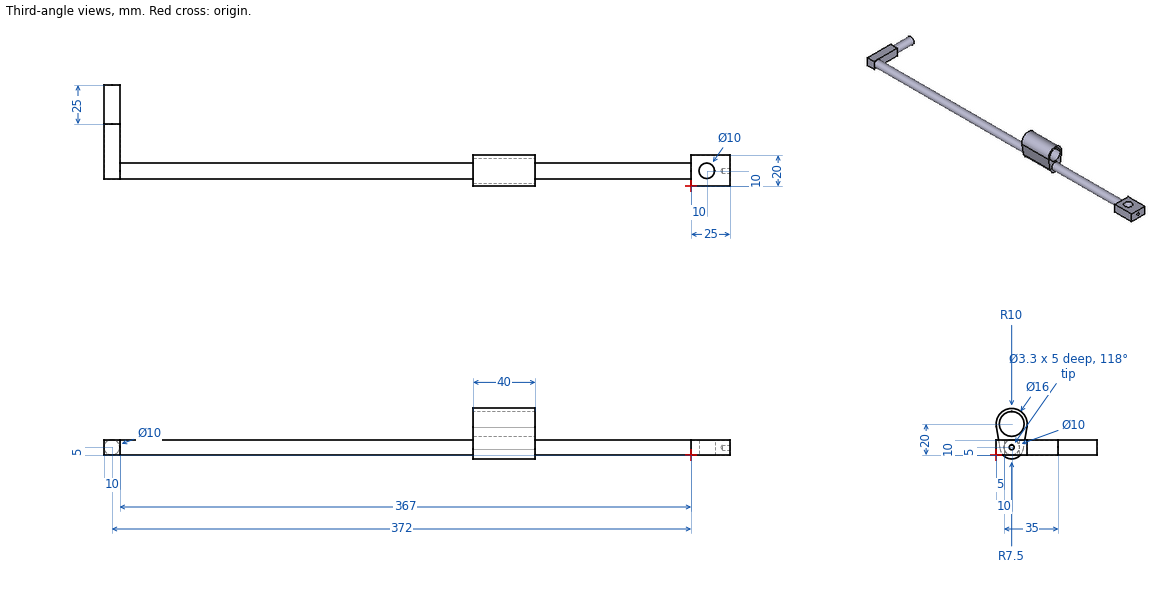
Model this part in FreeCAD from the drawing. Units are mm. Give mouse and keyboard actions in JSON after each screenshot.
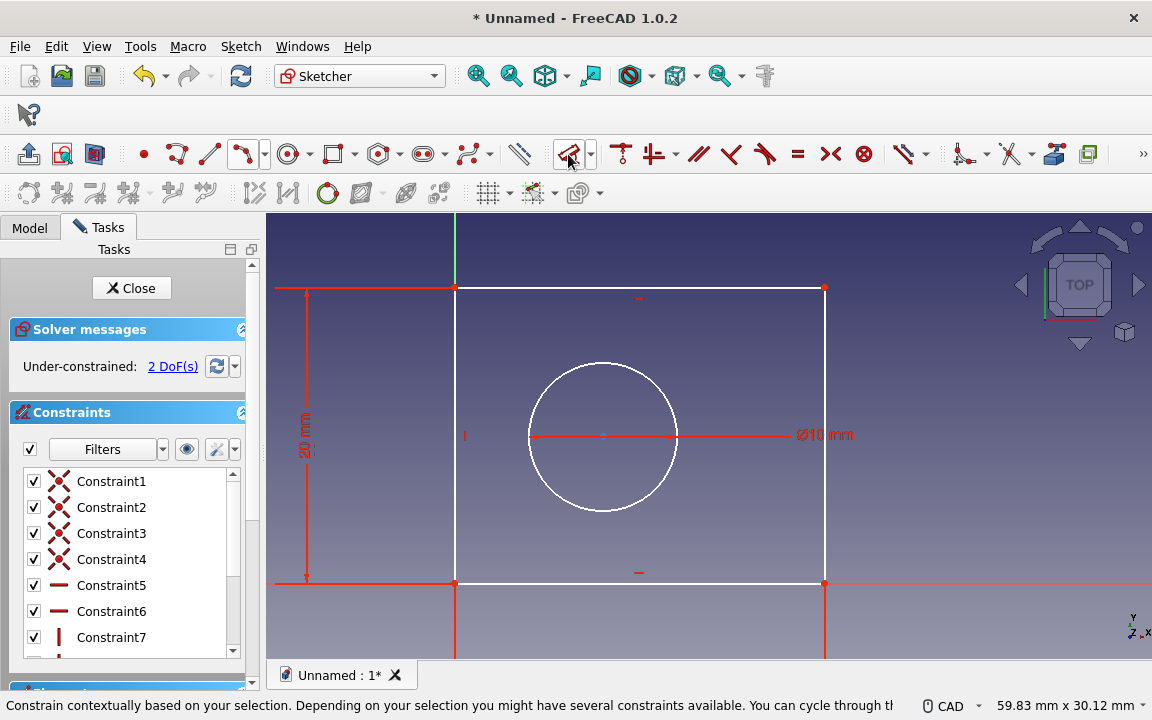
{"action": "left_click", "coordinate": [603, 437]}
{"action": "left_click", "coordinate": [529, 618]}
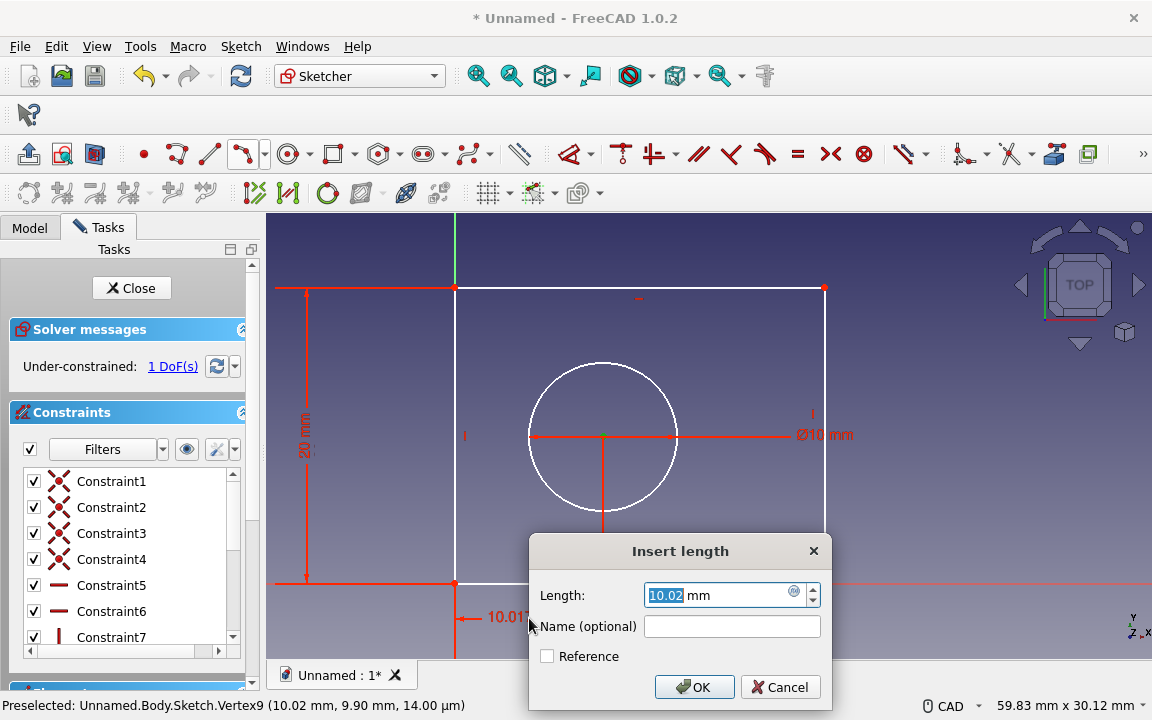
{"action": "type", "text": "10"}
{"action": "key", "text": "Return"}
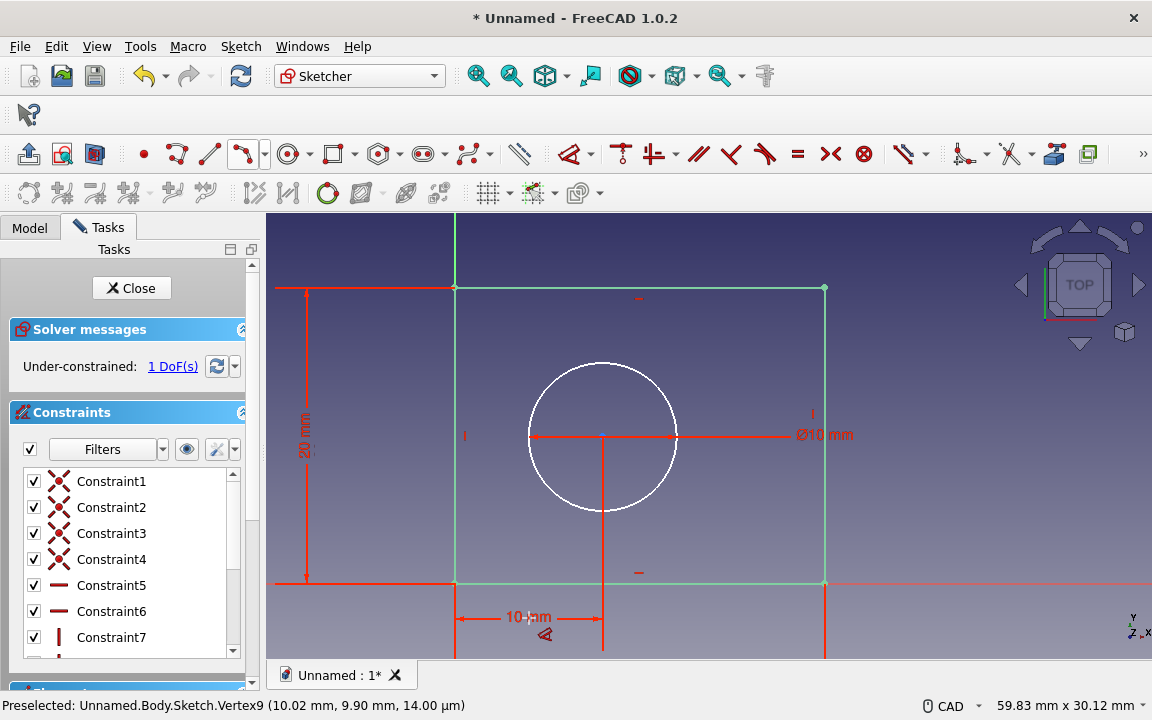
{"action": "left_click", "coordinate": [603, 437]}
{"action": "left_click", "coordinate": [421, 510]}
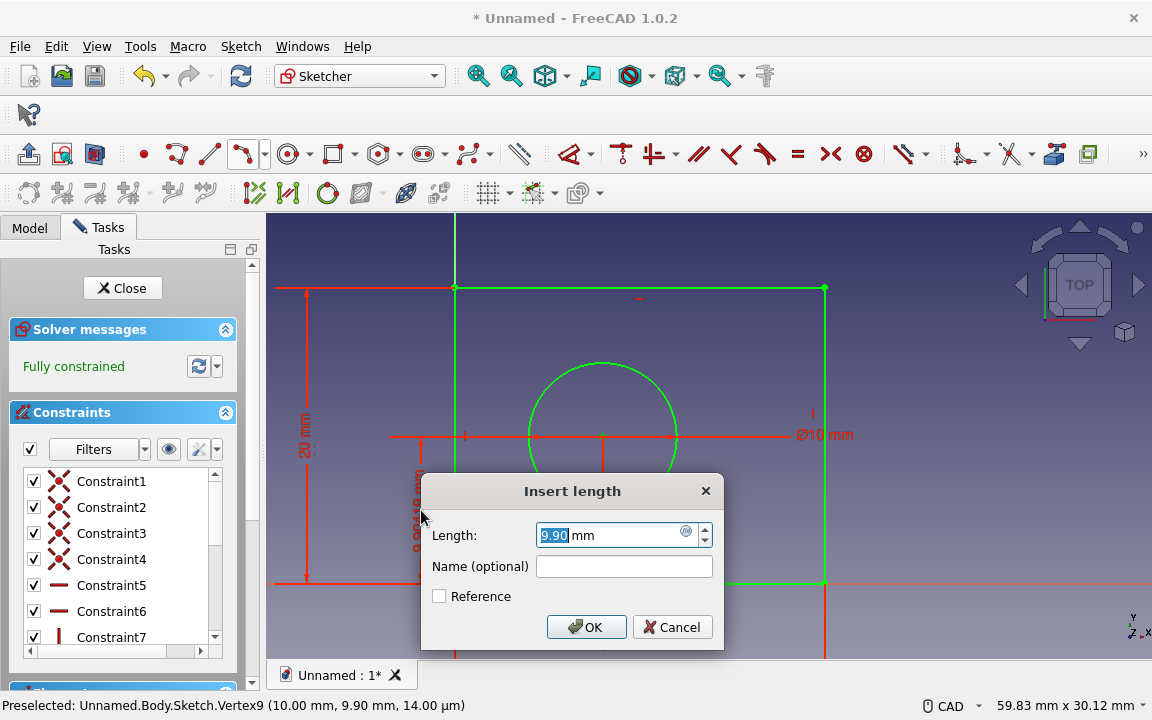
{"action": "type", "text": "10"}
{"action": "key", "text": "Return"}
{"action": "key", "text": "Escape"}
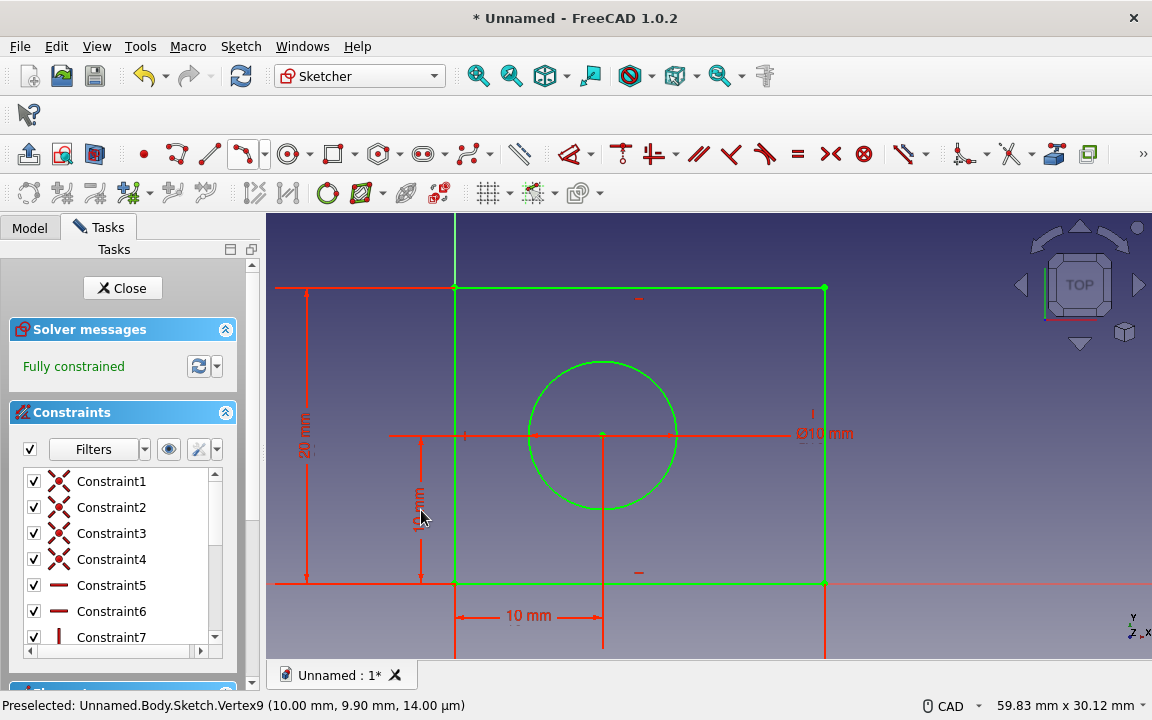
{"action": "left_click", "coordinate": [123, 288]}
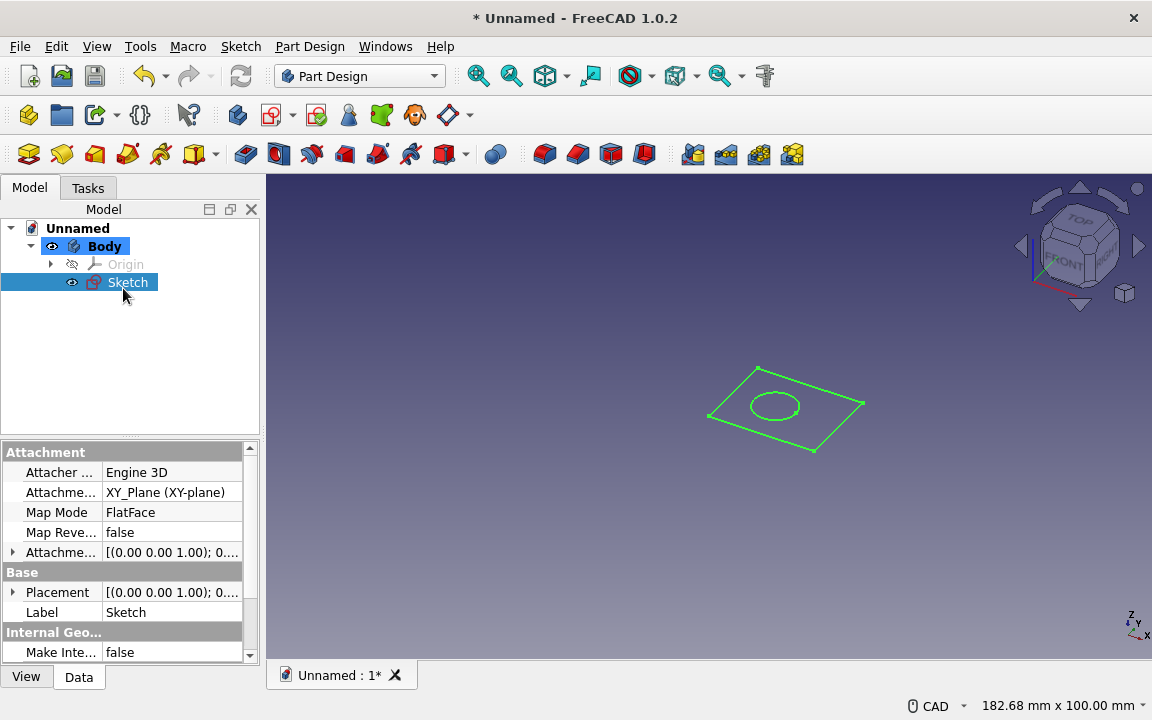
{"action": "left_click", "coordinate": [29, 154]}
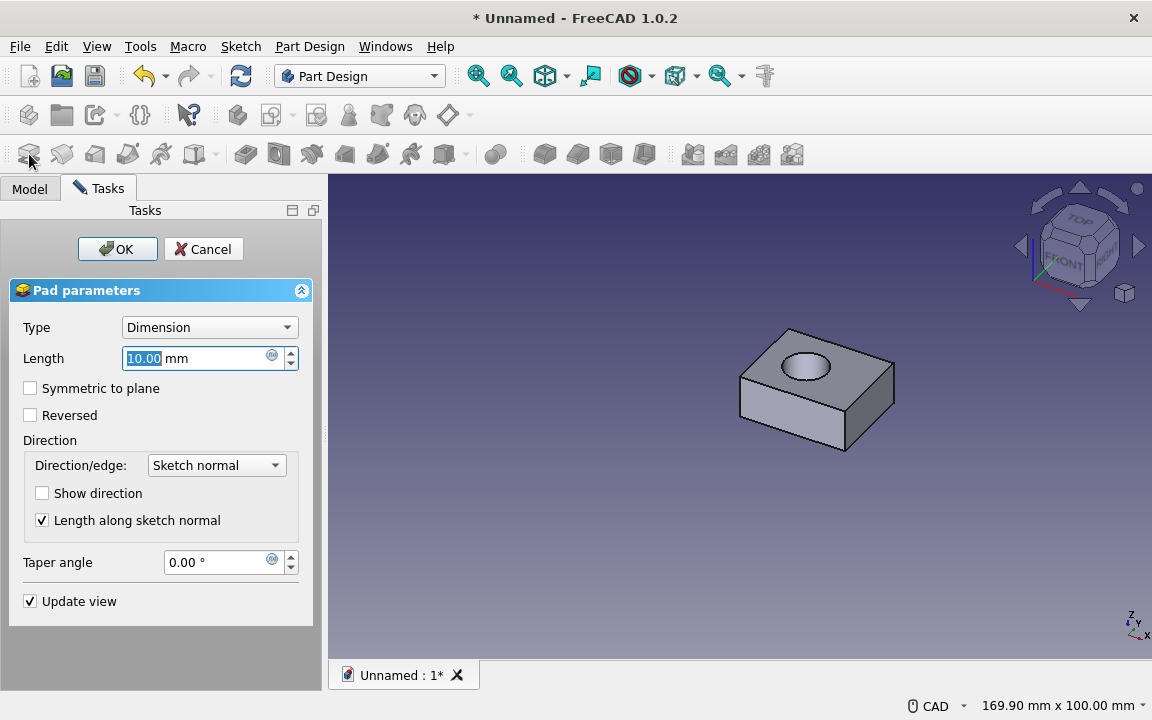
{"action": "type", "text": "10"}
{"action": "key", "text": "Tab"}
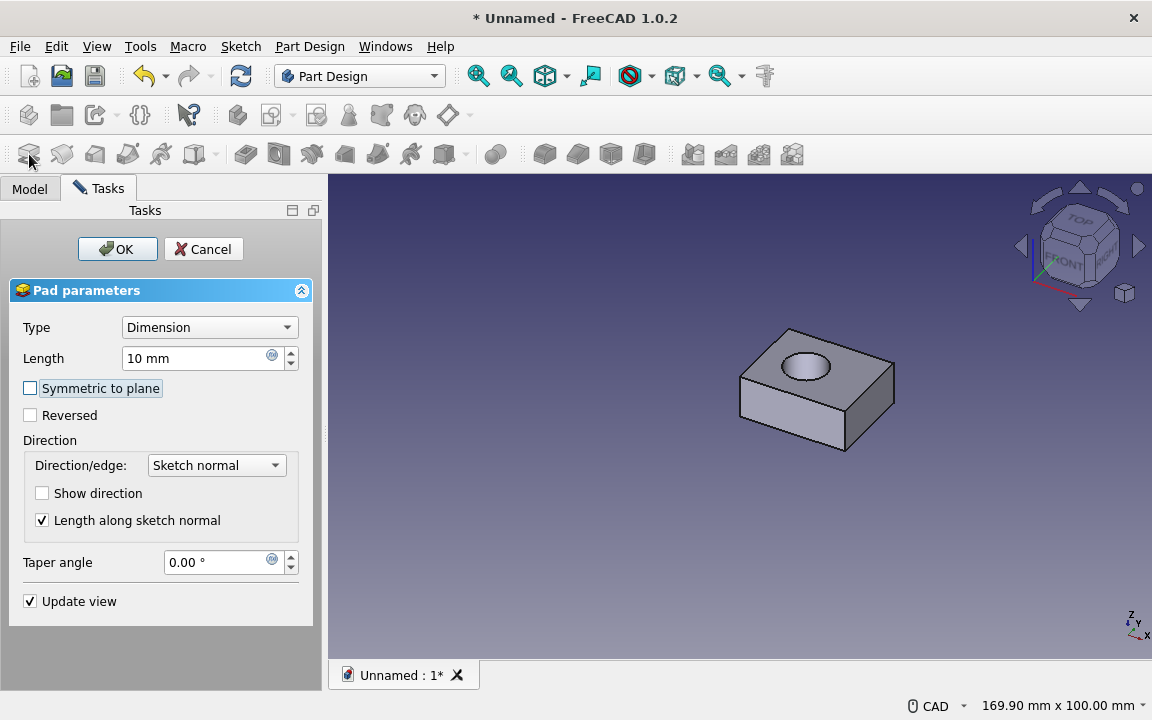
{"action": "left_click", "coordinate": [118, 249]}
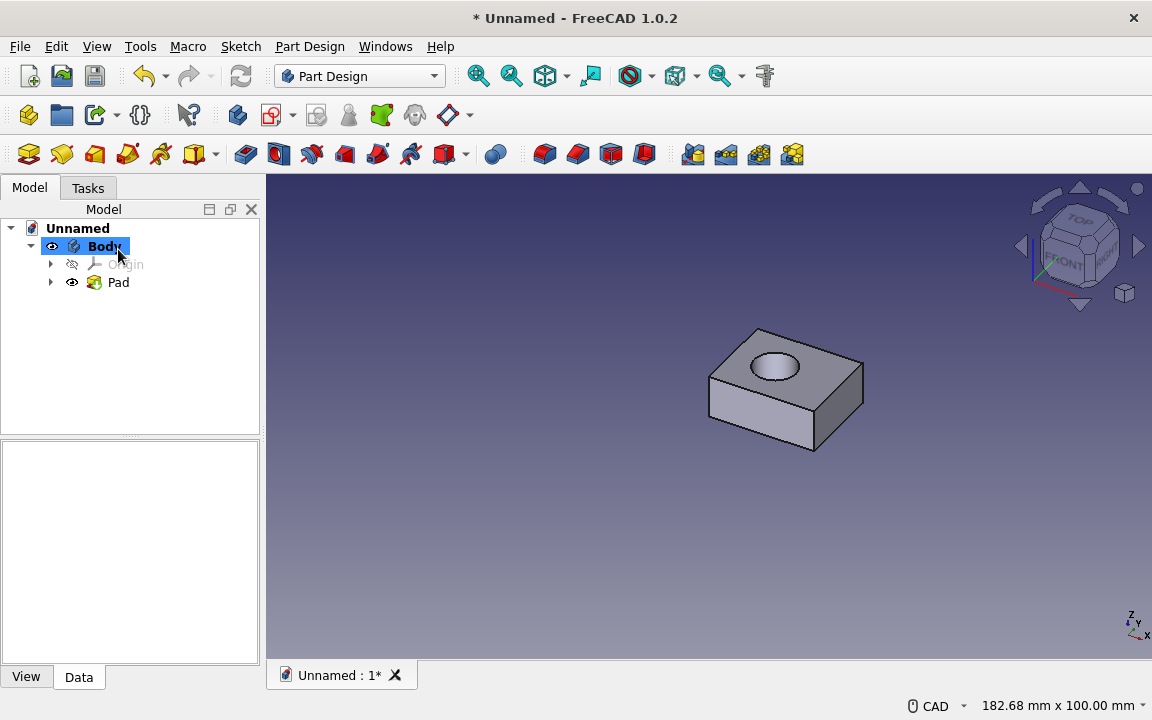
{"action": "left_click", "coordinate": [479, 76]}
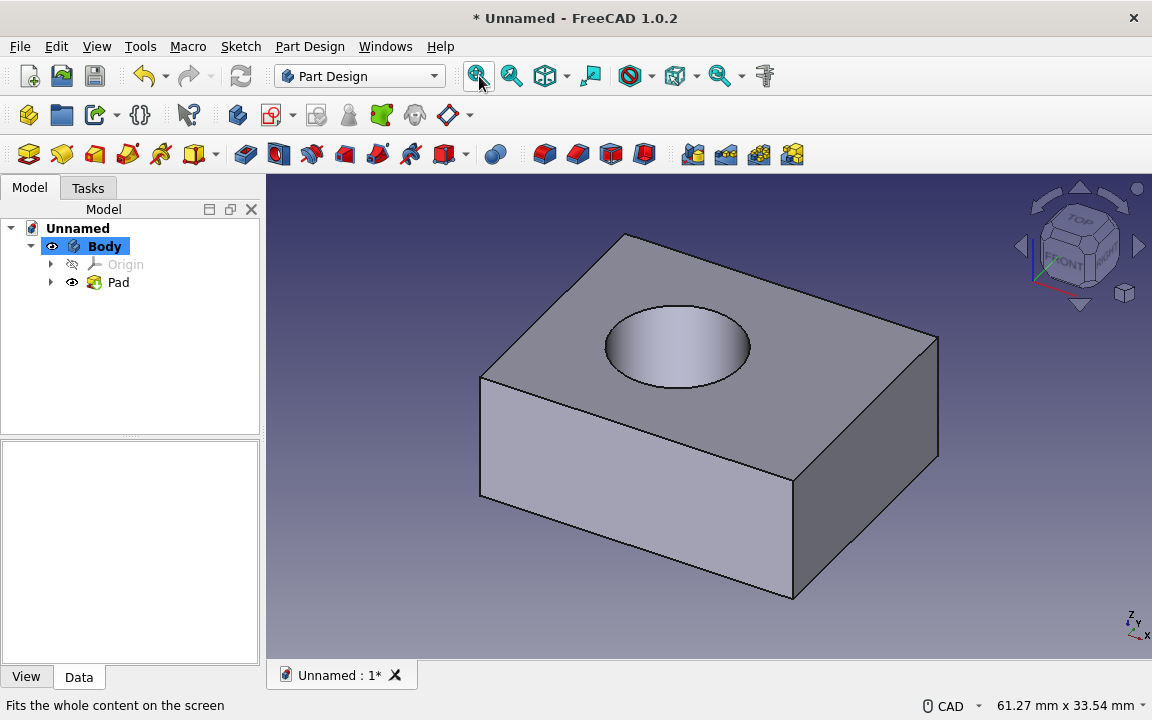
{"action": "left_click", "coordinate": [270, 116]}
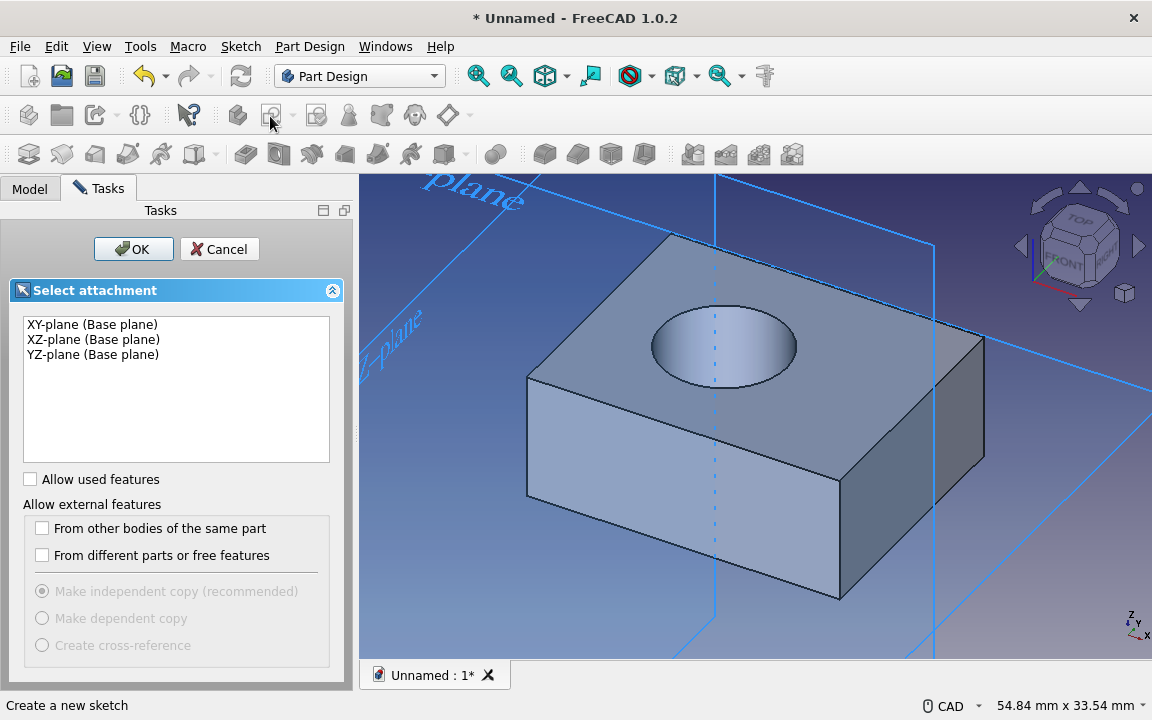
{"action": "left_click", "coordinate": [84, 354]}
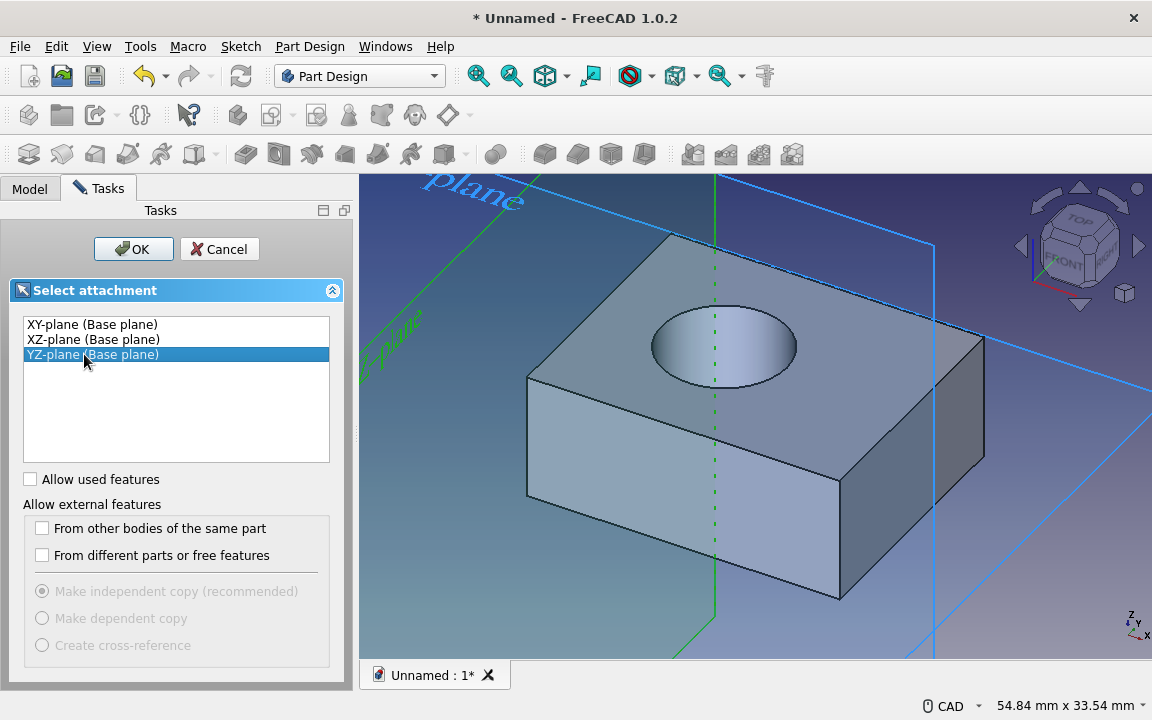
{"action": "left_click", "coordinate": [134, 249]}